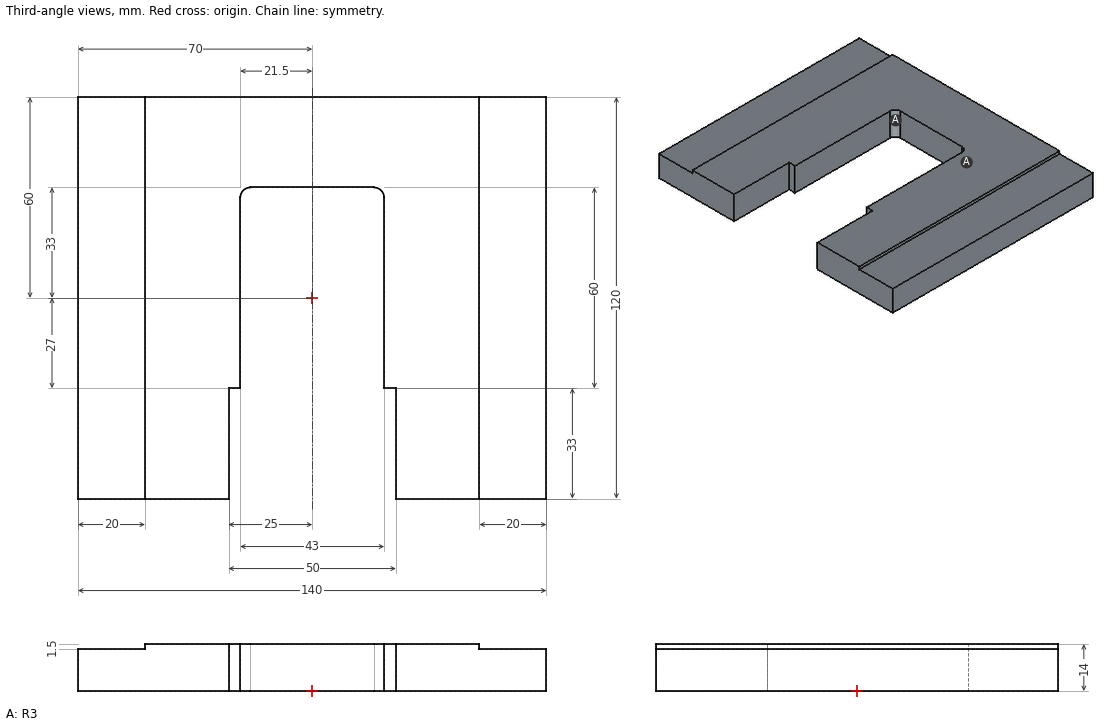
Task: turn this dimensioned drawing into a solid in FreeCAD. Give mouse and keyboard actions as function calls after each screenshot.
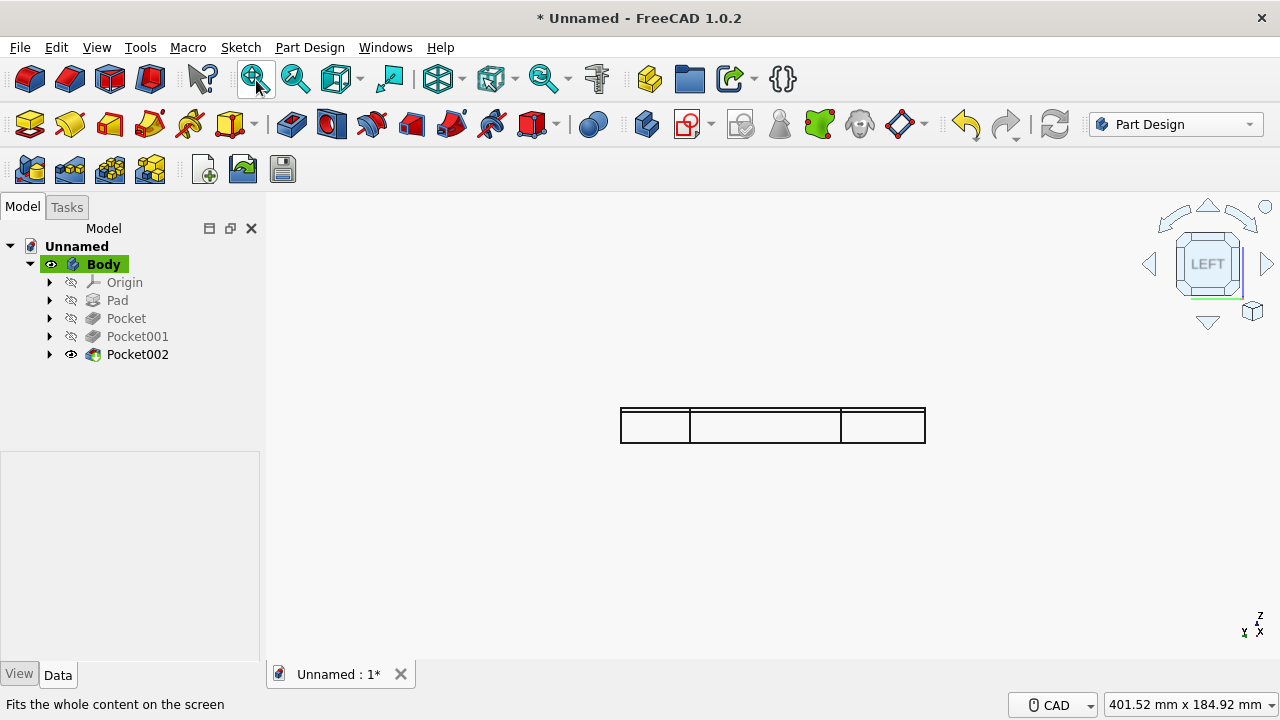
key(0)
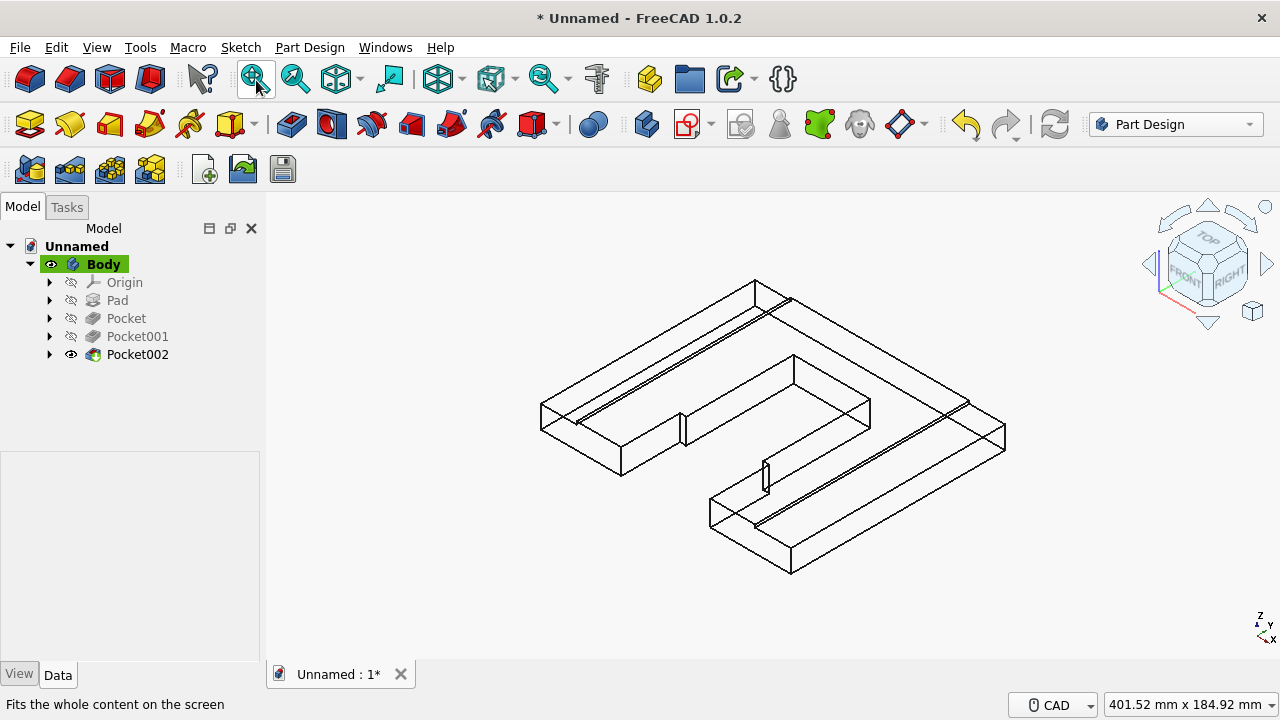
click(794, 368)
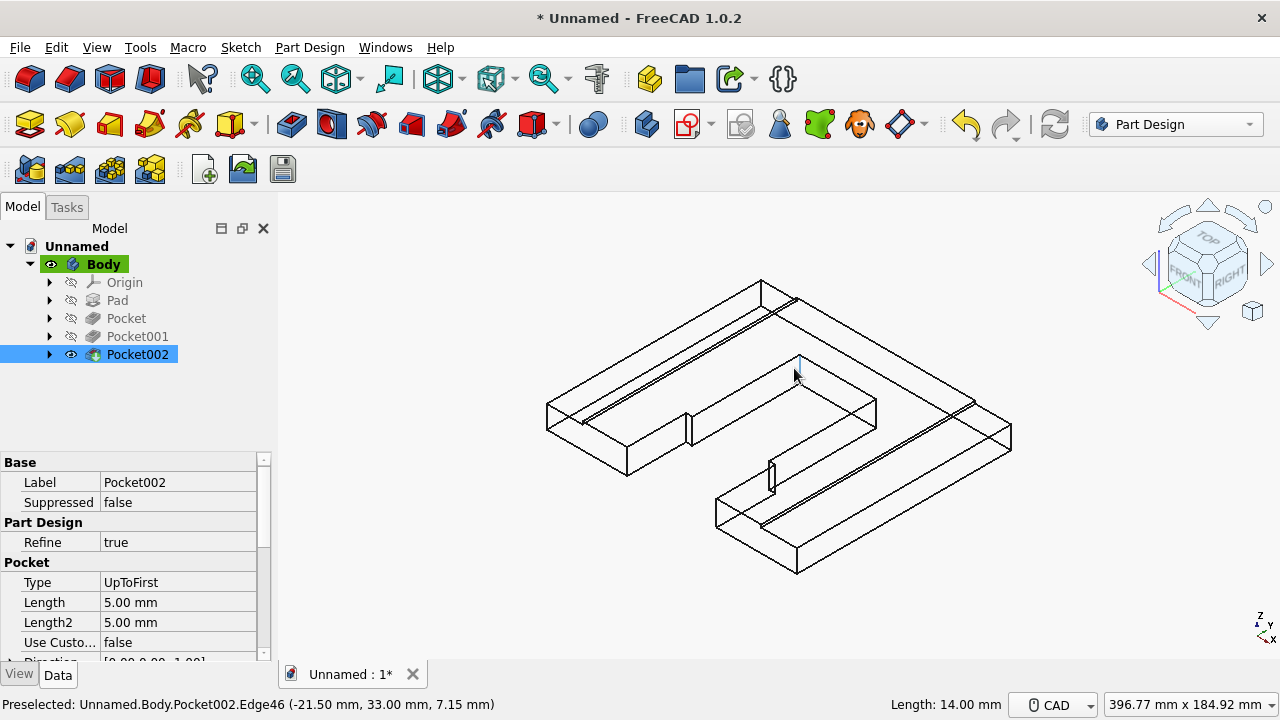
click(876, 413, ctrl)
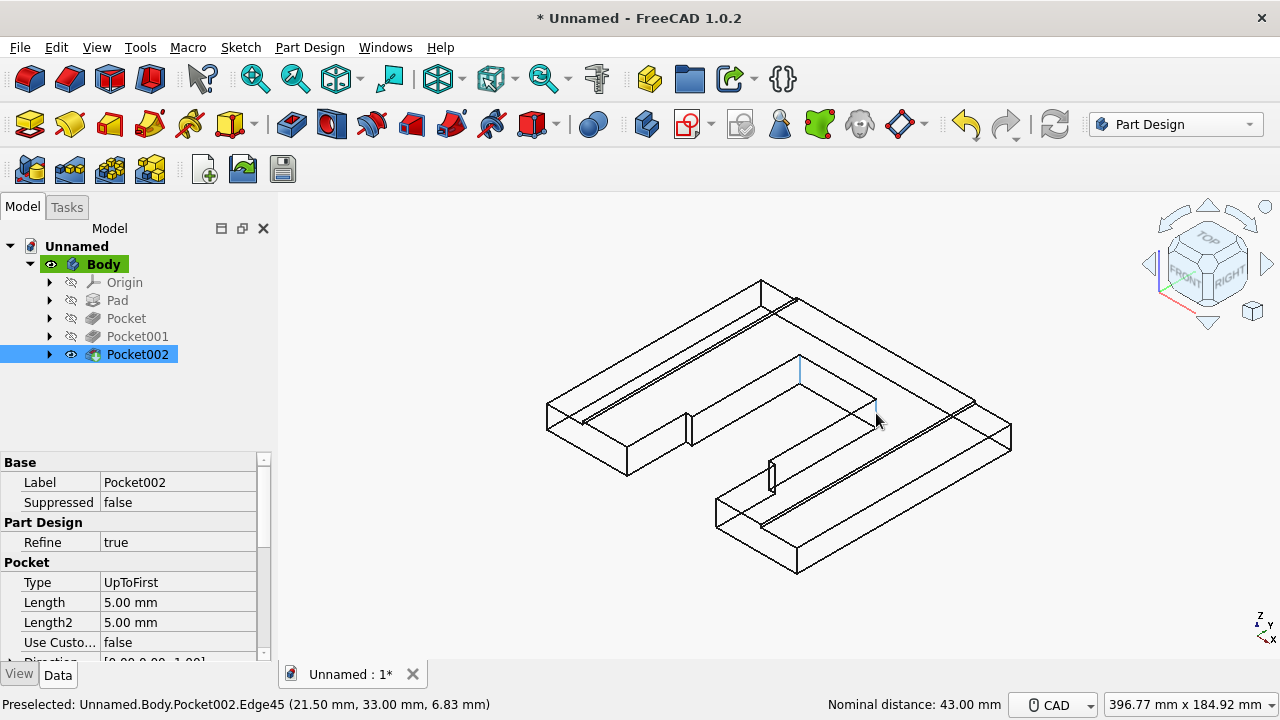
key(v)
key(1)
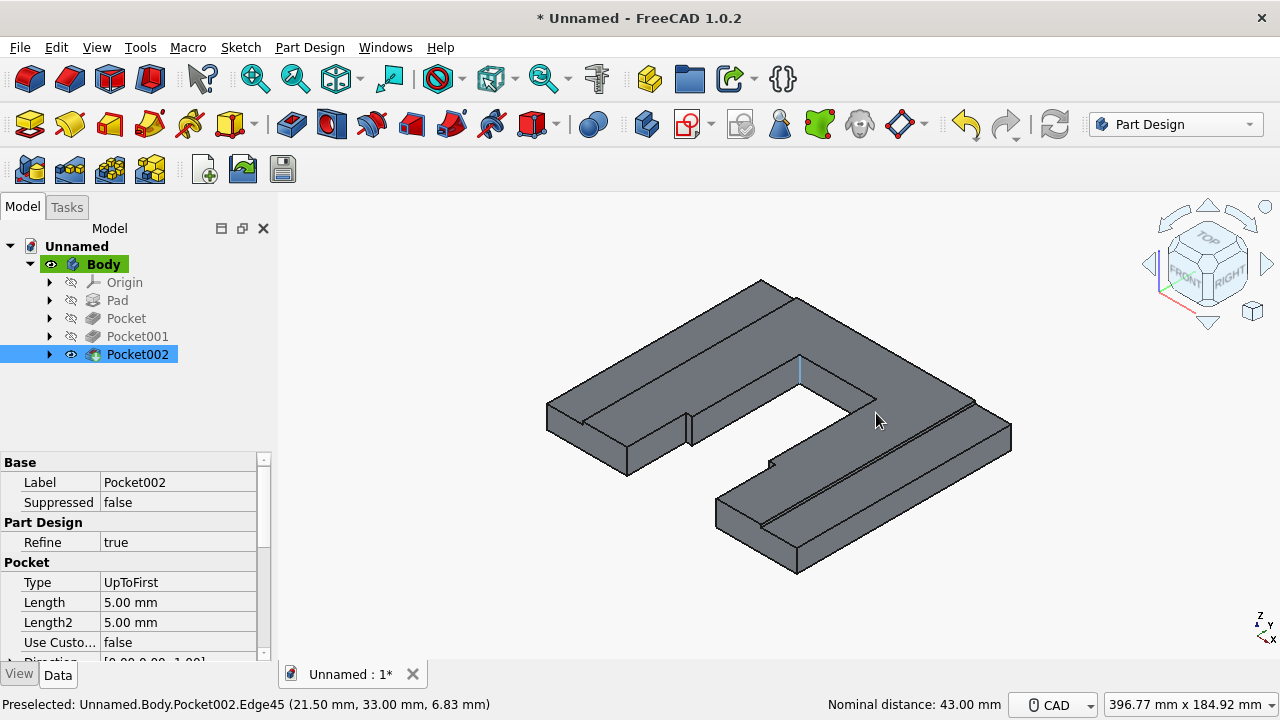
click(30, 80)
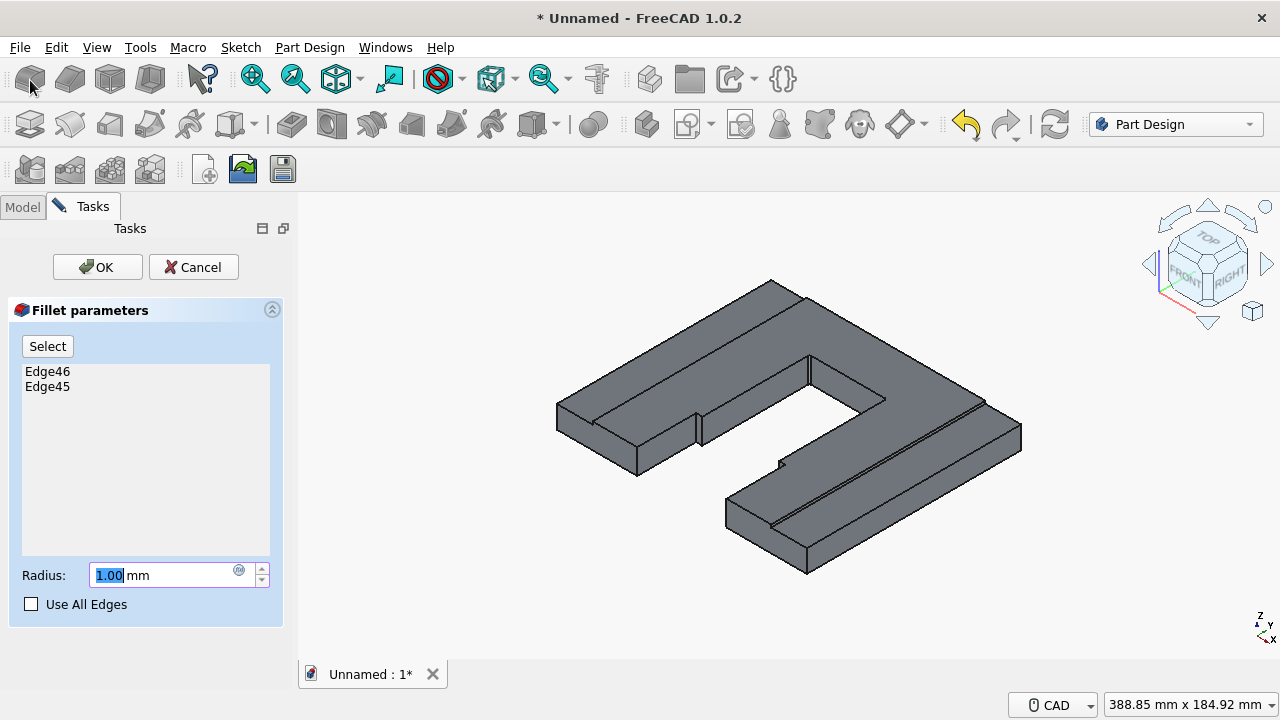
text(3)
key(Tab)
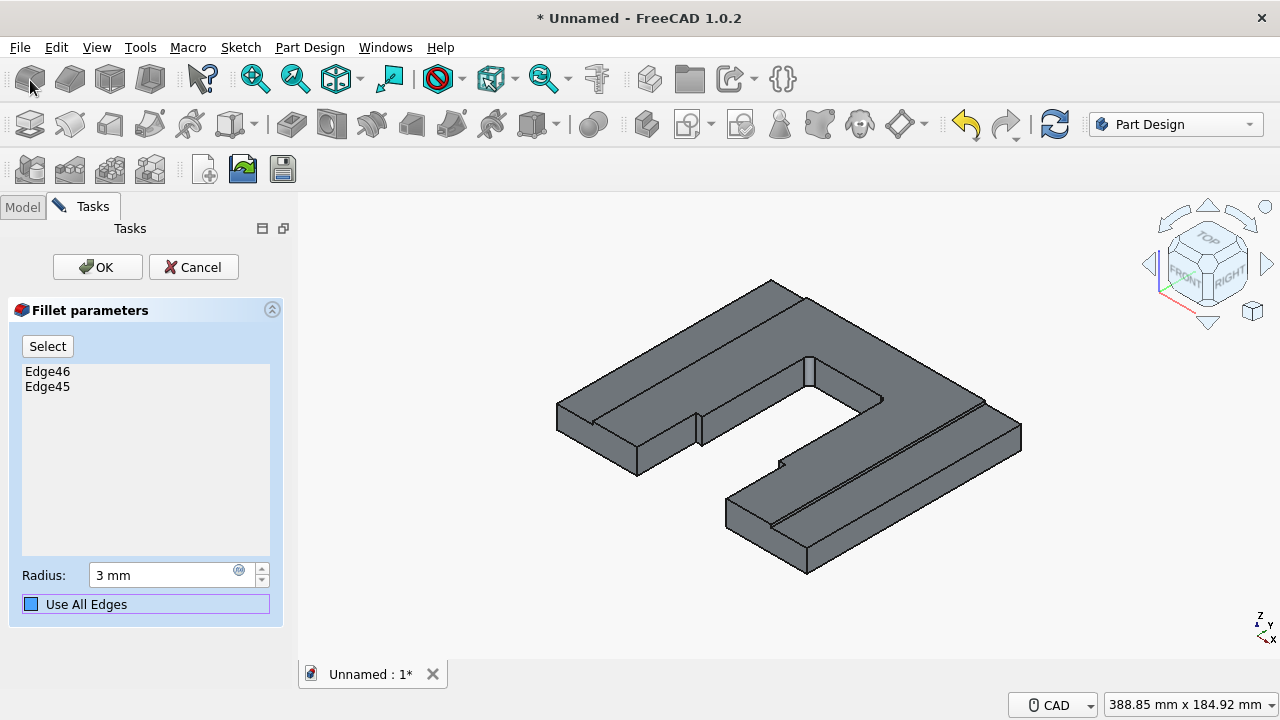
click(98, 267)